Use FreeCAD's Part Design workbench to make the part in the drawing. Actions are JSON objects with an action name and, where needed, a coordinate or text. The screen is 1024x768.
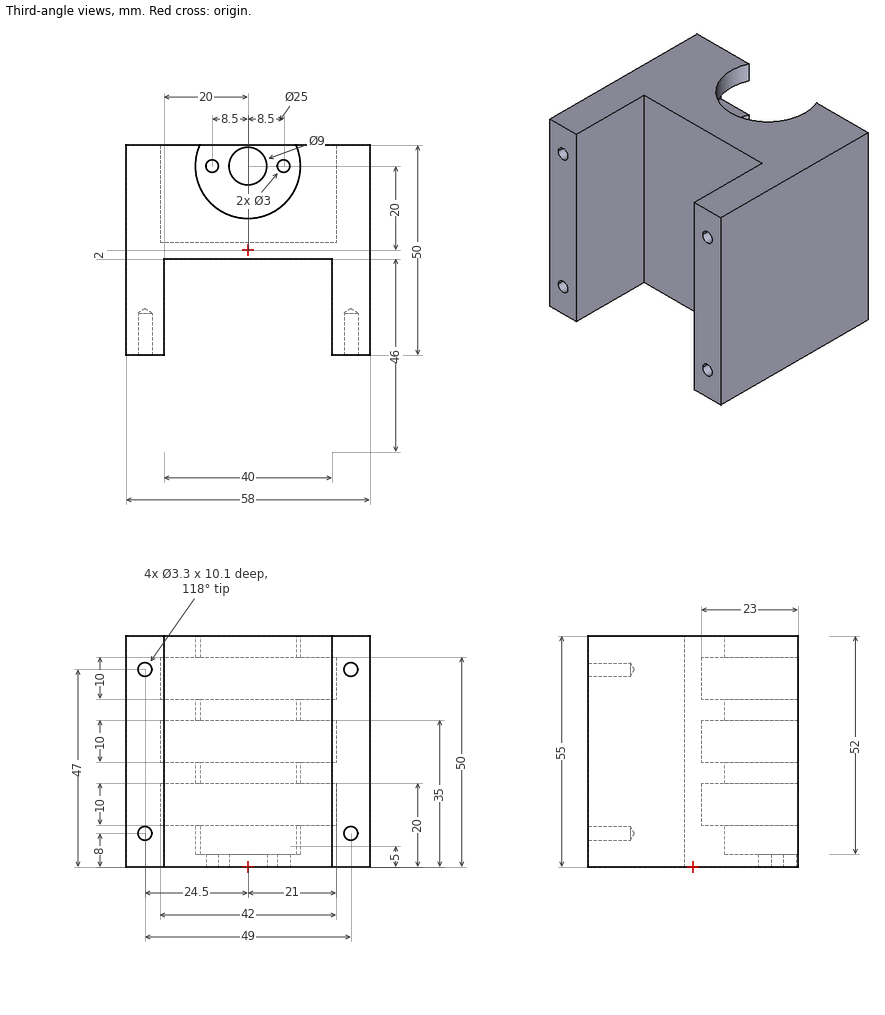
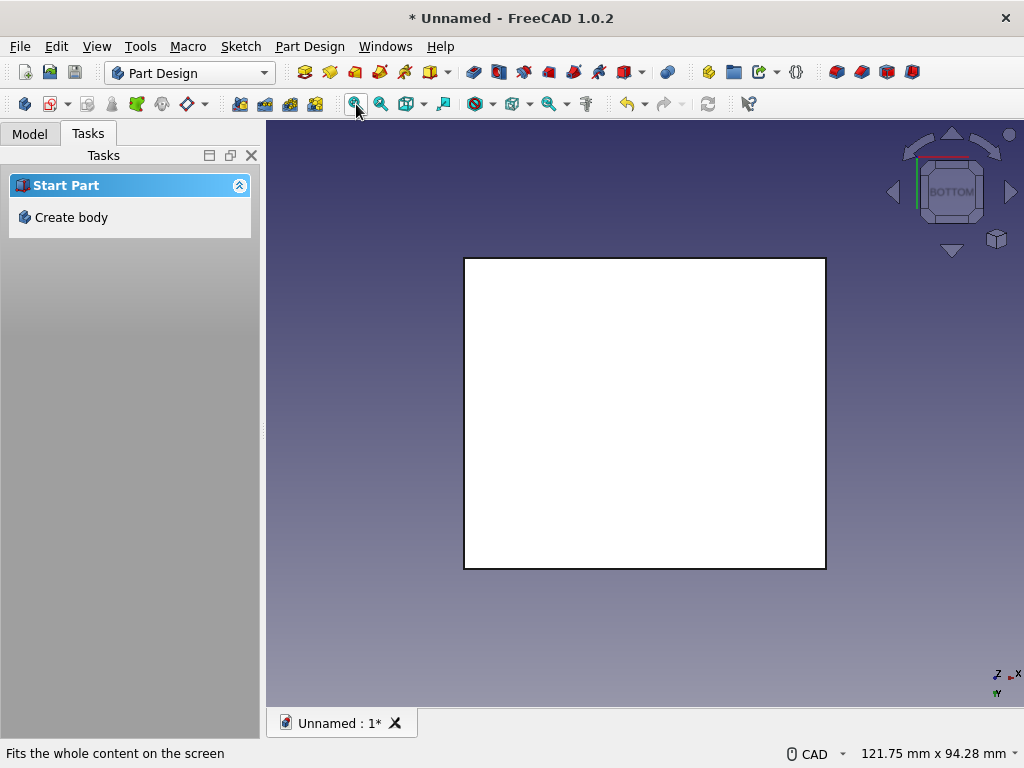
{"action": "left_click", "coordinate": [645, 412]}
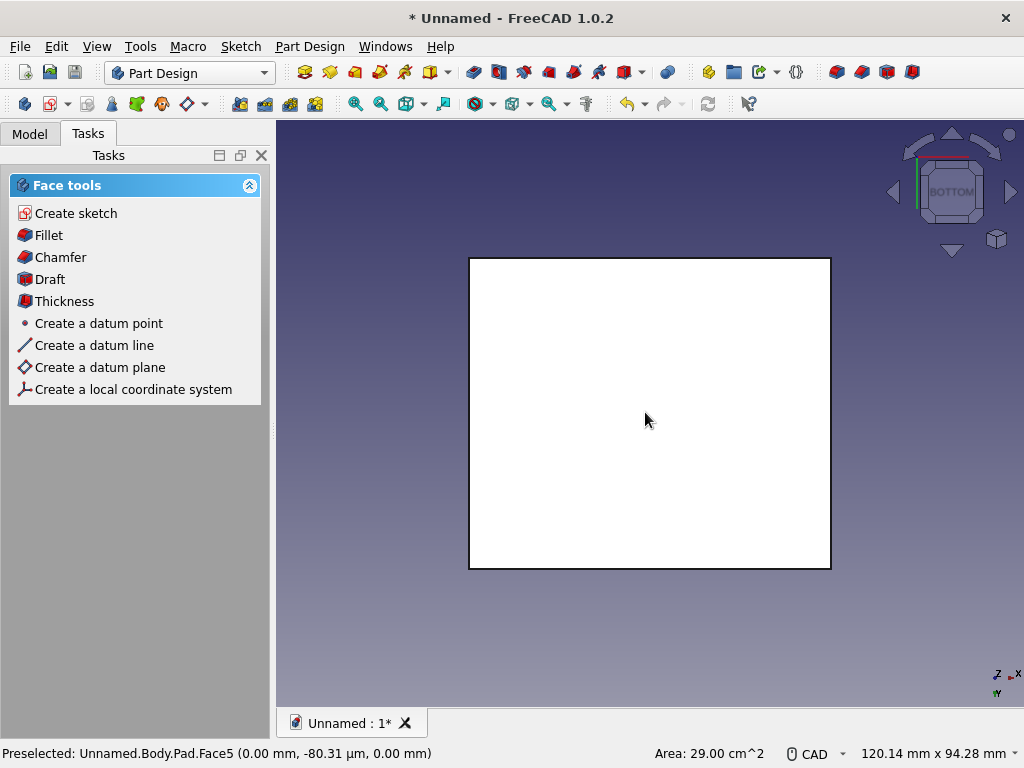
{"action": "left_click", "coordinate": [50, 104]}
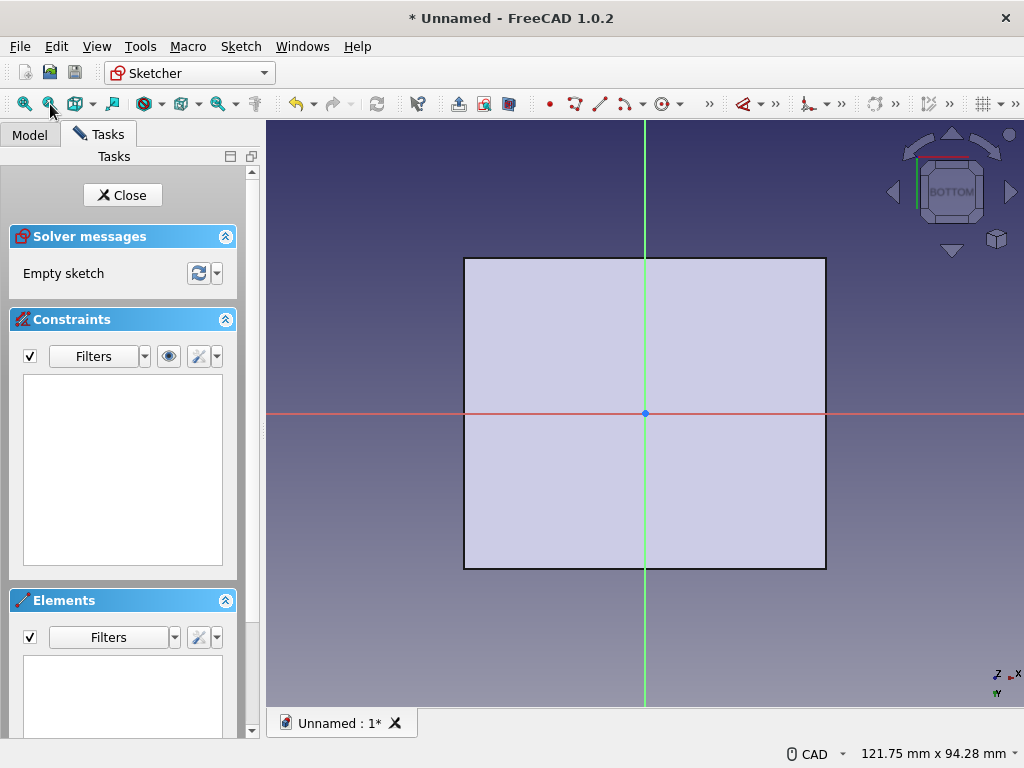
{"action": "scroll", "coordinate": [701, 552], "scroll_direction": "up", "scroll_amount": 4}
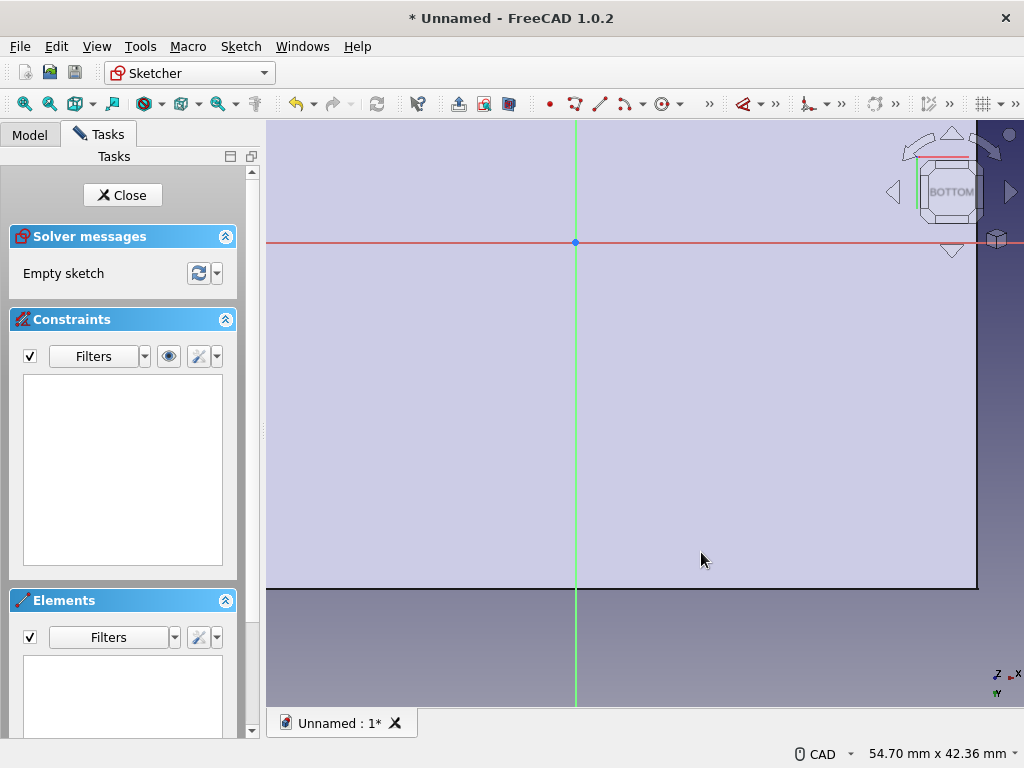
{"action": "key", "text": "g c"}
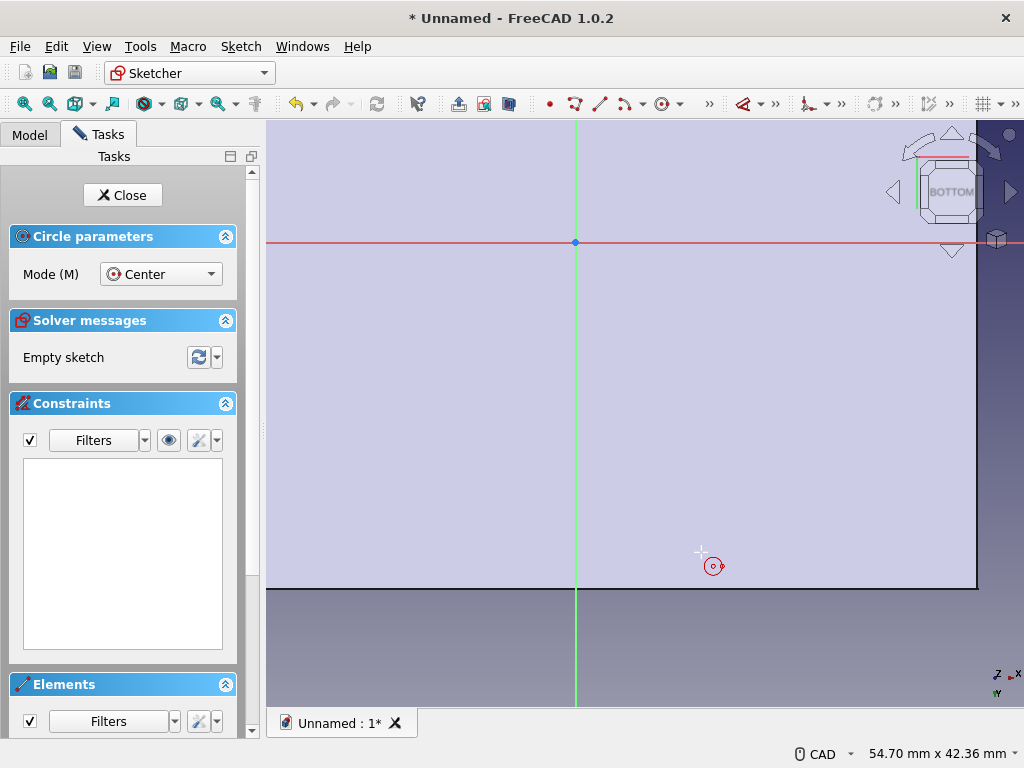
{"action": "left_click", "coordinate": [576, 520]}
{"action": "mouse_move", "coordinate": [620, 476]}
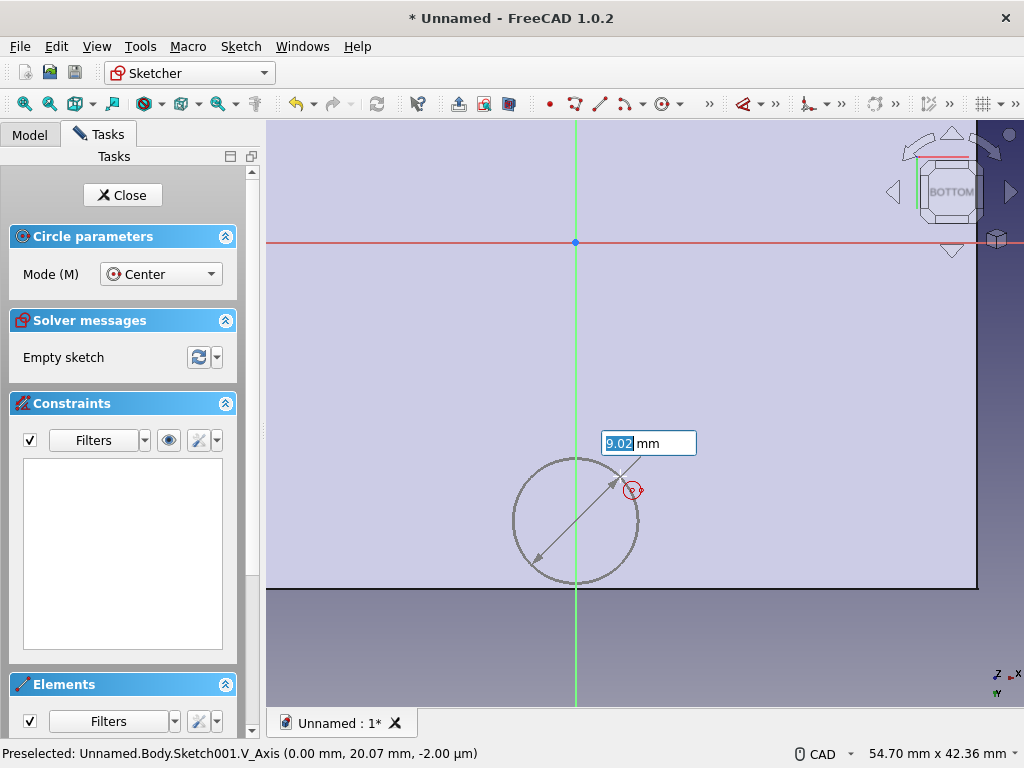
{"action": "type", "text": "9"}
{"action": "key", "text": "Return"}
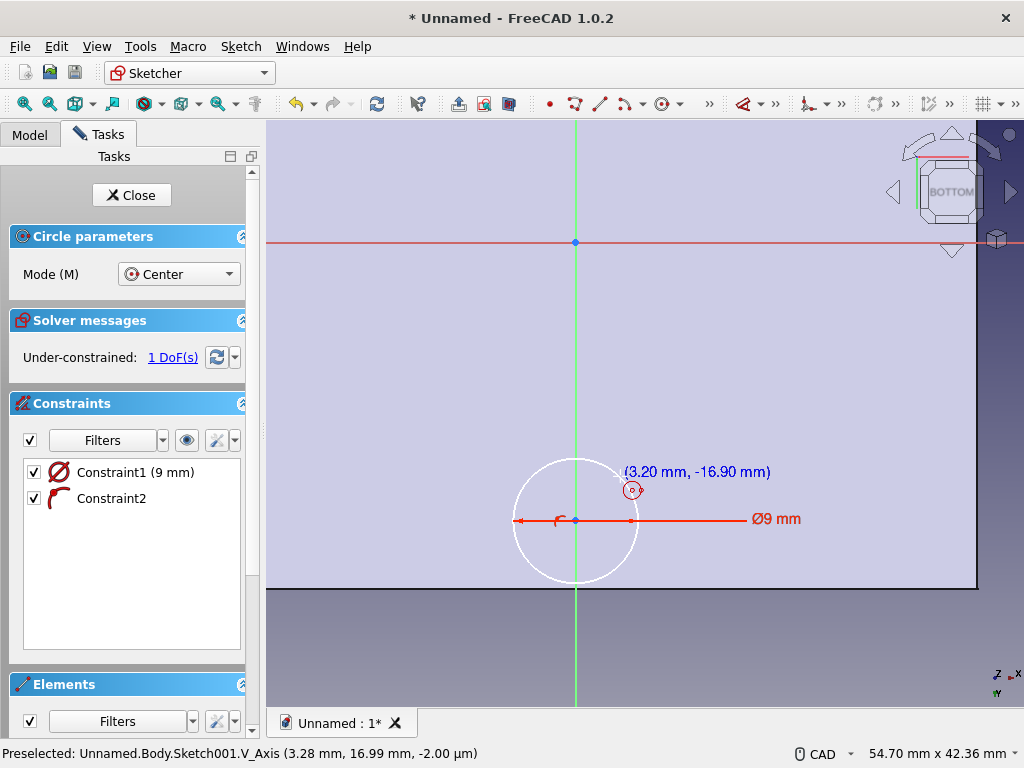
{"action": "left_click", "coordinate": [693, 520]}
{"action": "mouse_move", "coordinate": [708, 505]}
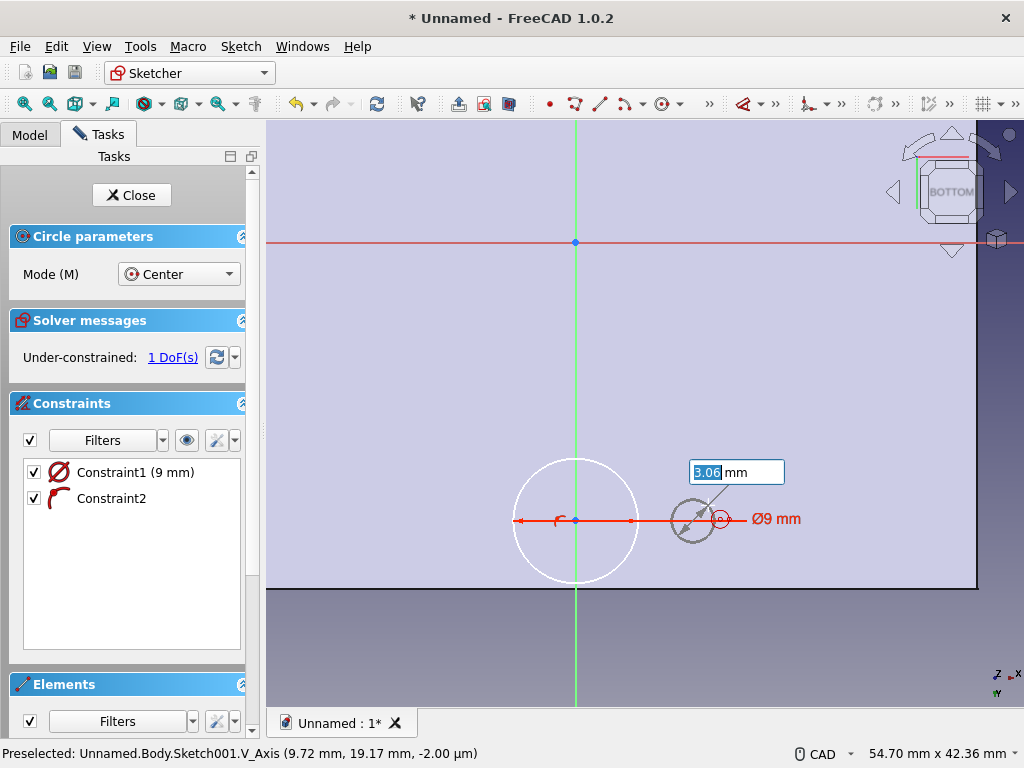
{"action": "type", "text": "3"}
{"action": "key", "text": "Return"}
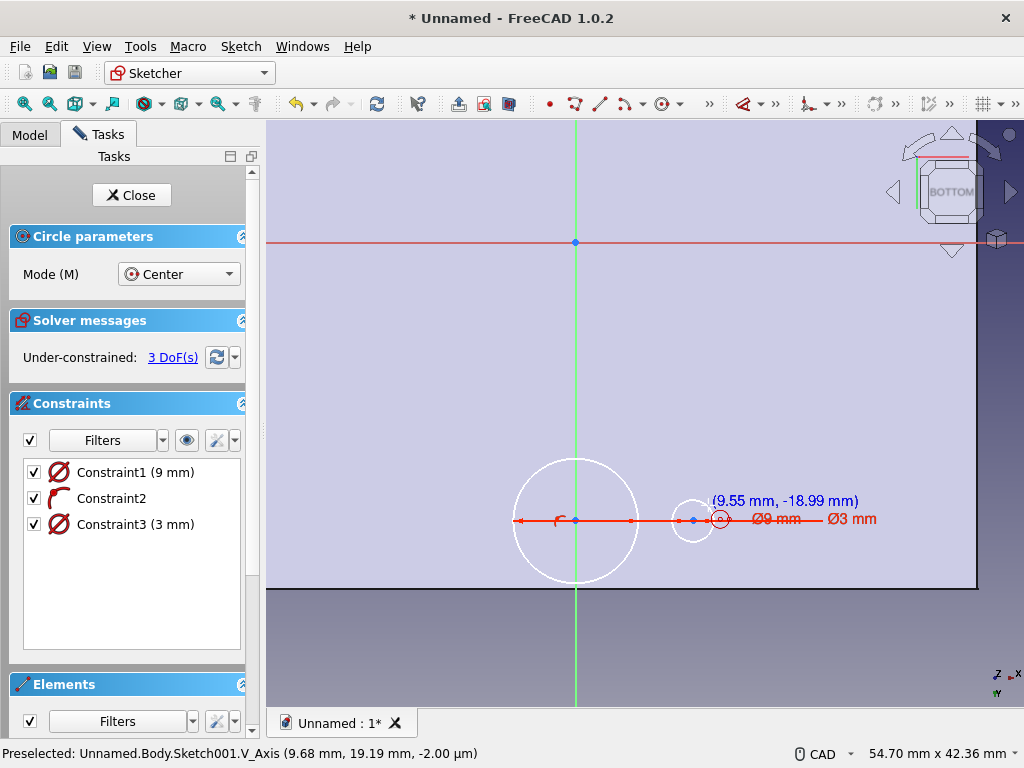
{"action": "left_click", "coordinate": [458, 520]}
{"action": "mouse_move", "coordinate": [473, 505]}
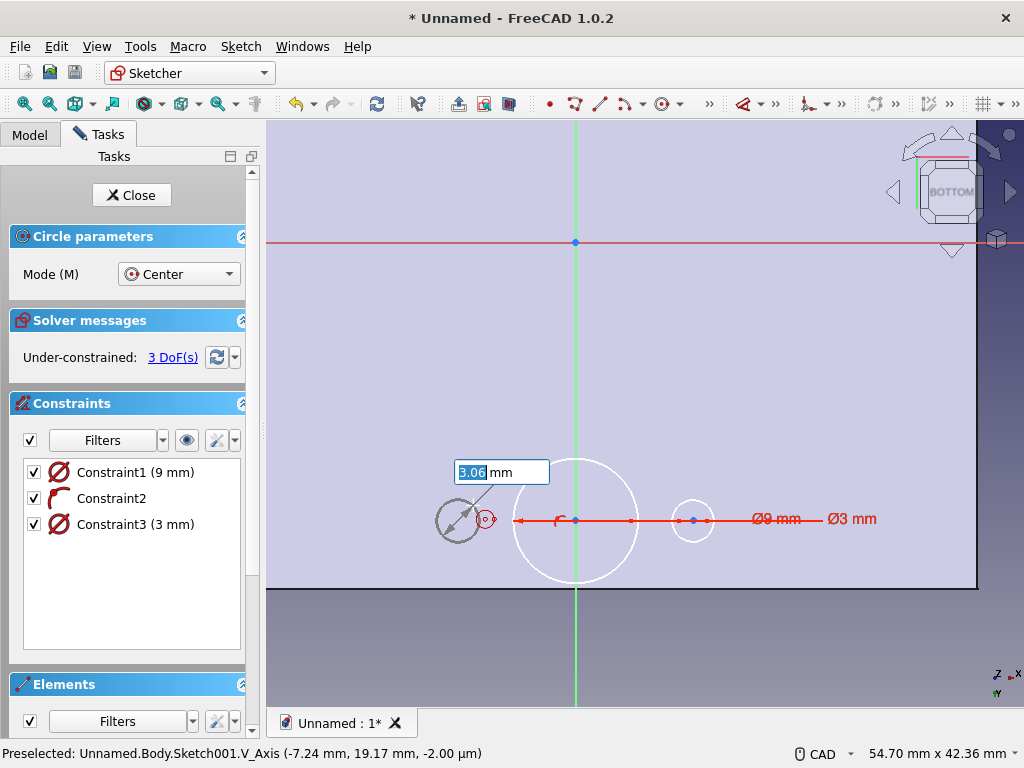
{"action": "type", "text": "3"}
{"action": "key", "text": "Return"}
{"action": "key", "text": "Escape"}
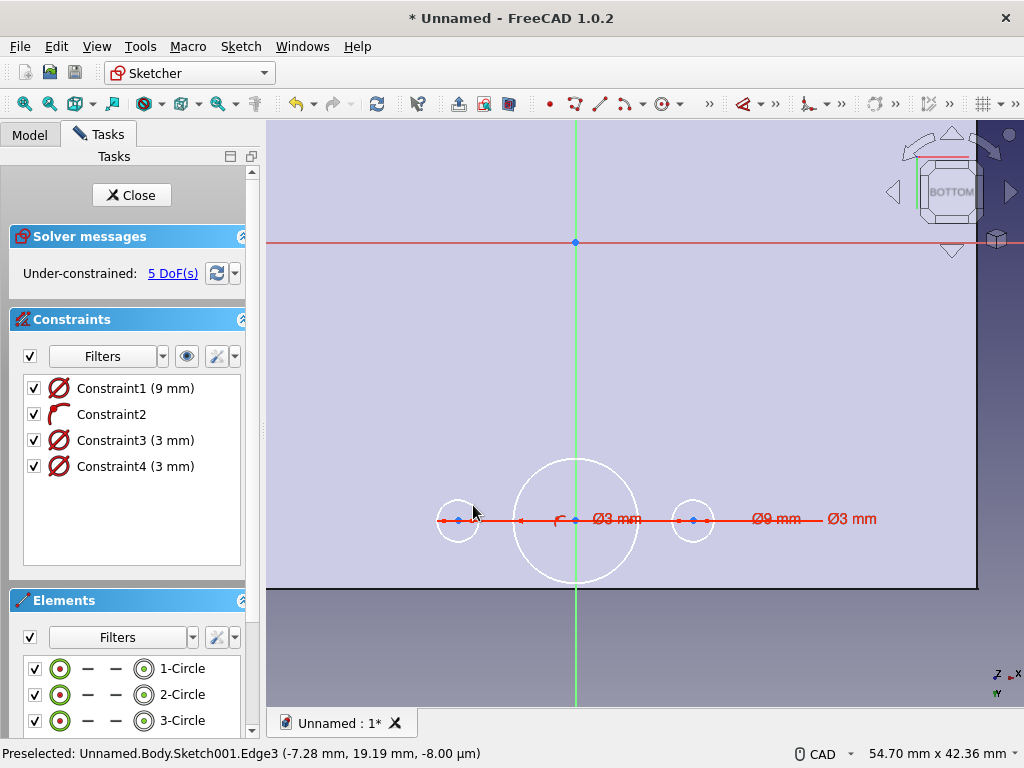
{"action": "left_click", "coordinate": [742, 104]}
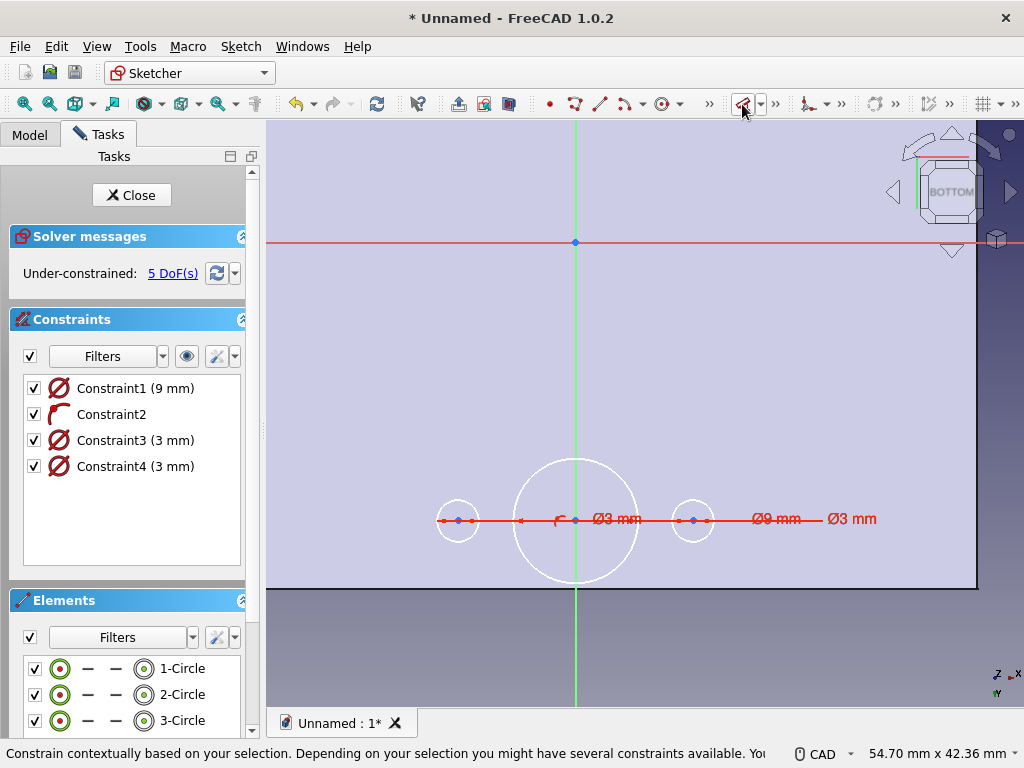
{"action": "left_click", "coordinate": [576, 521]}
{"action": "left_click", "coordinate": [610, 382]}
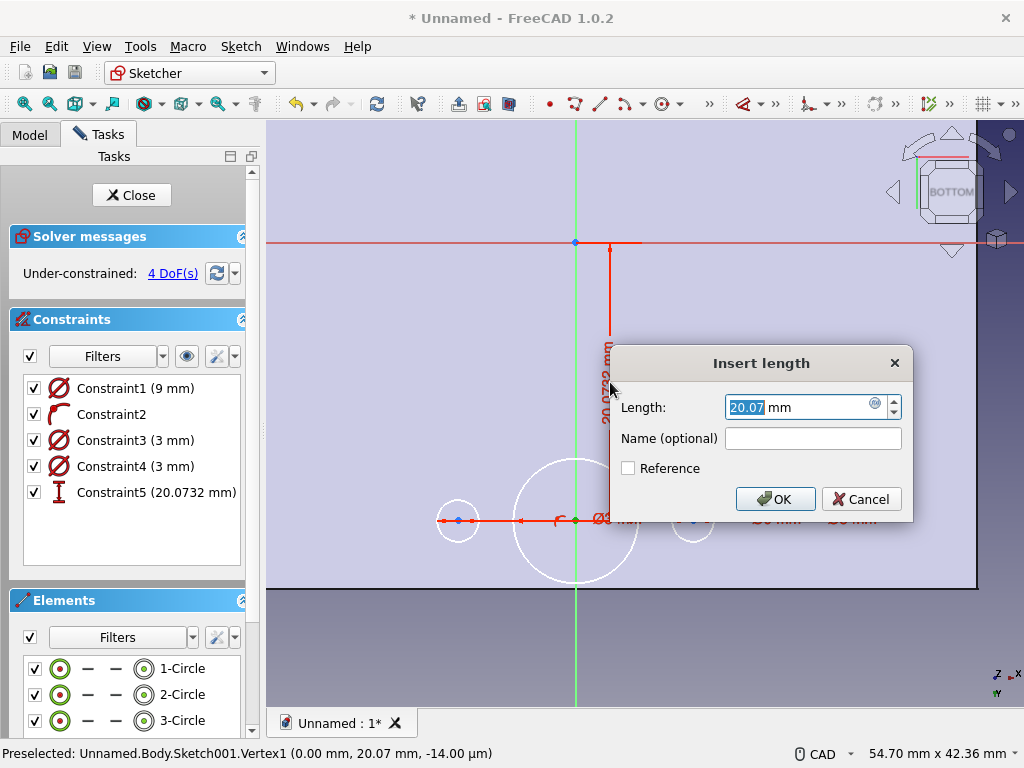
{"action": "type", "text": "20"}
{"action": "key", "text": "Return"}